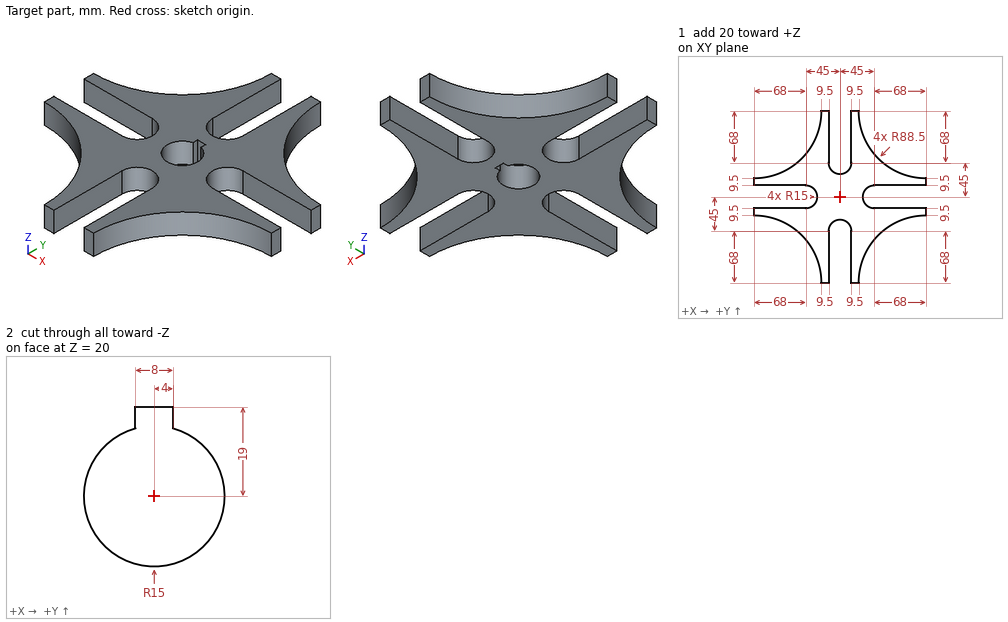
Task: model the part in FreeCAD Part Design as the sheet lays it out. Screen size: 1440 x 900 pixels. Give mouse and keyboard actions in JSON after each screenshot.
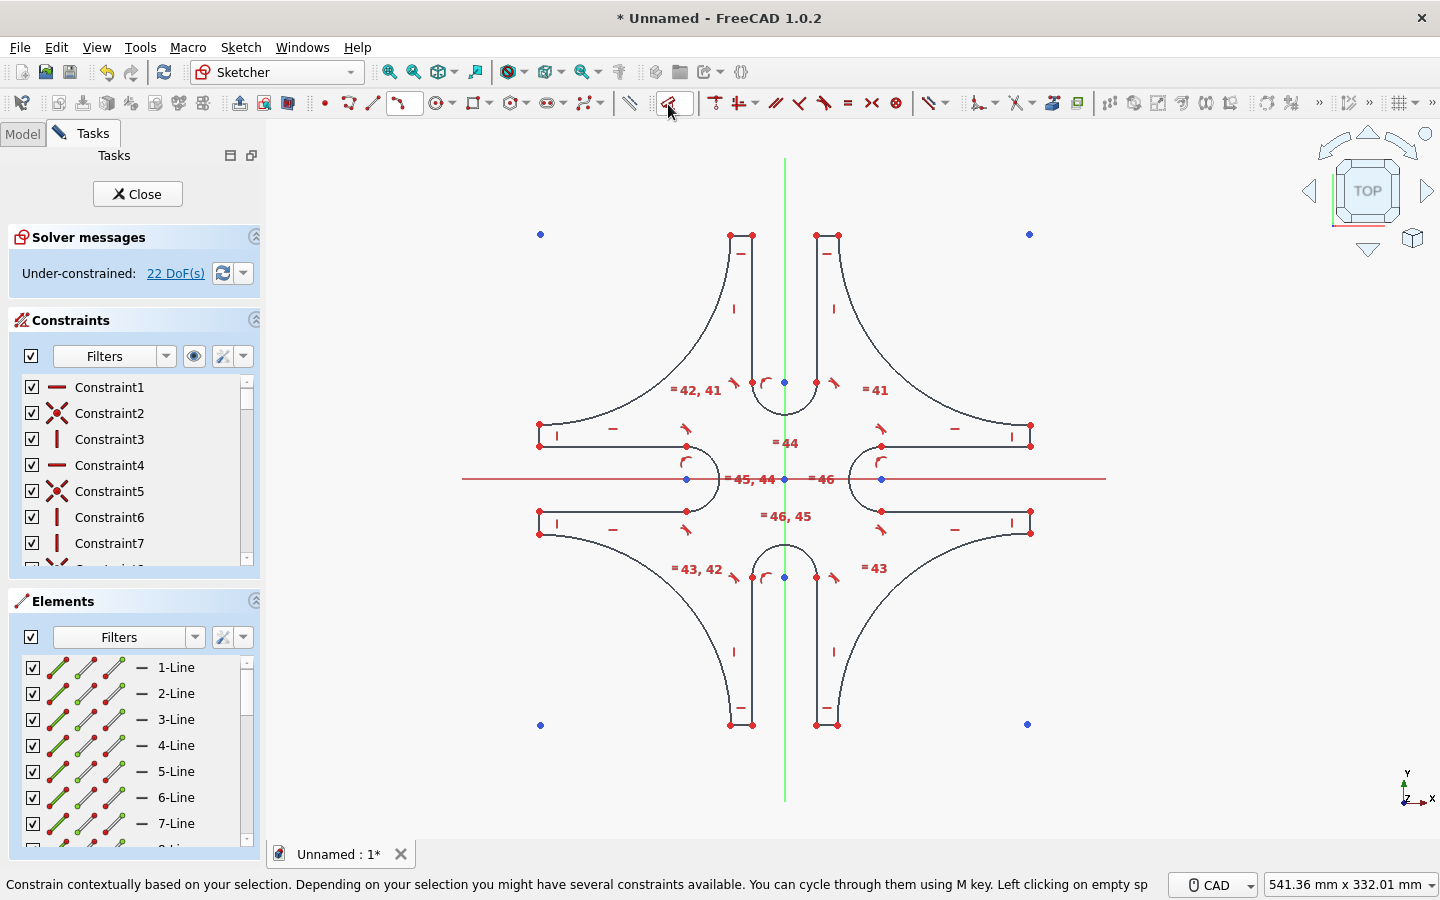
{"action": "left_click", "coordinate": [860, 322]}
{"action": "left_click", "coordinate": [832, 337]}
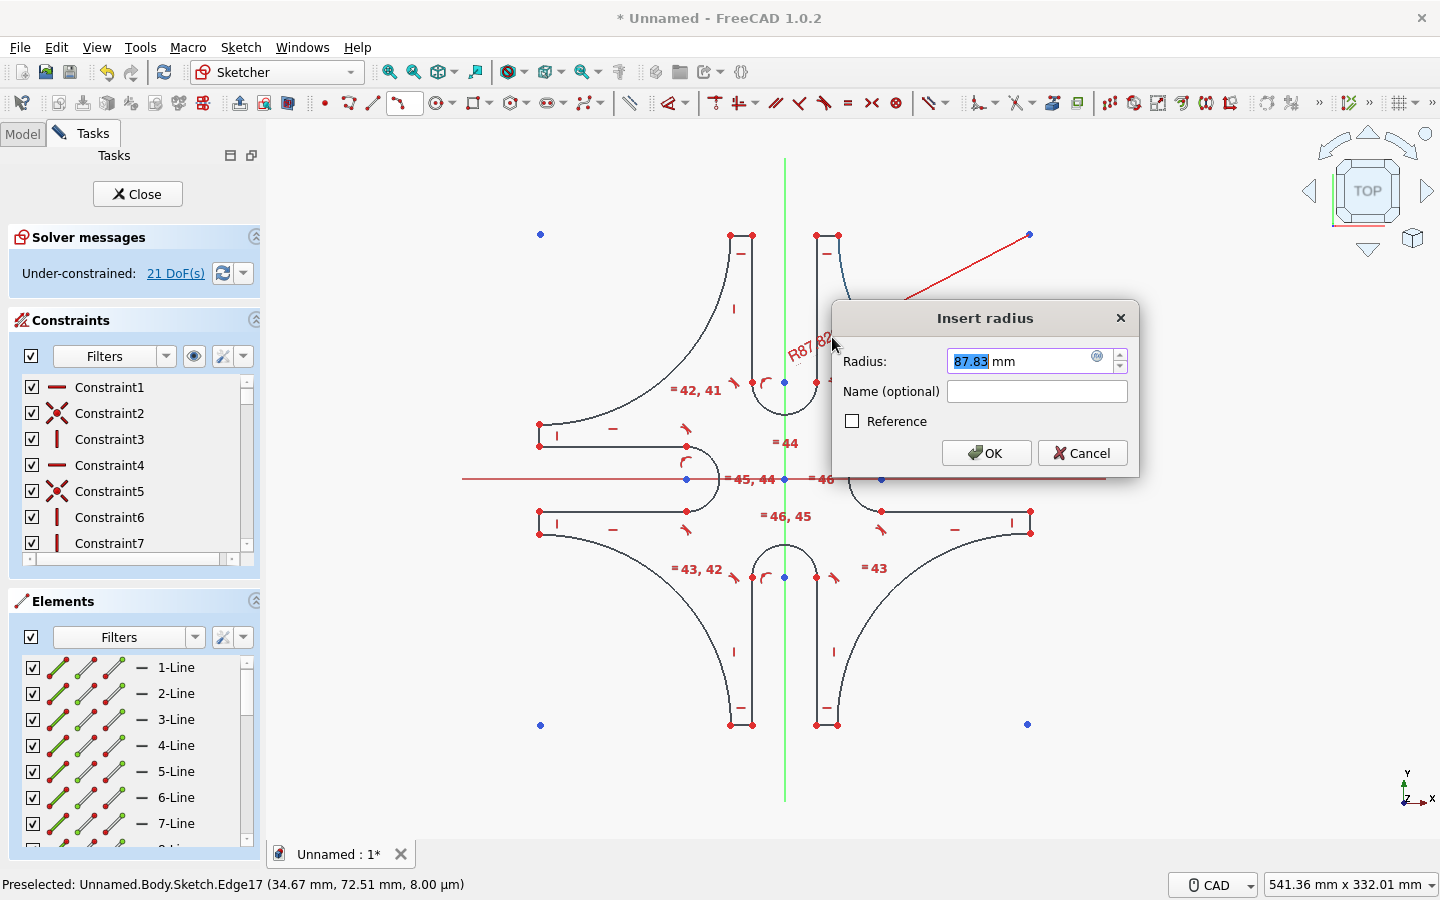
{"action": "type", "text": "88.5"}
{"action": "key", "text": "Return"}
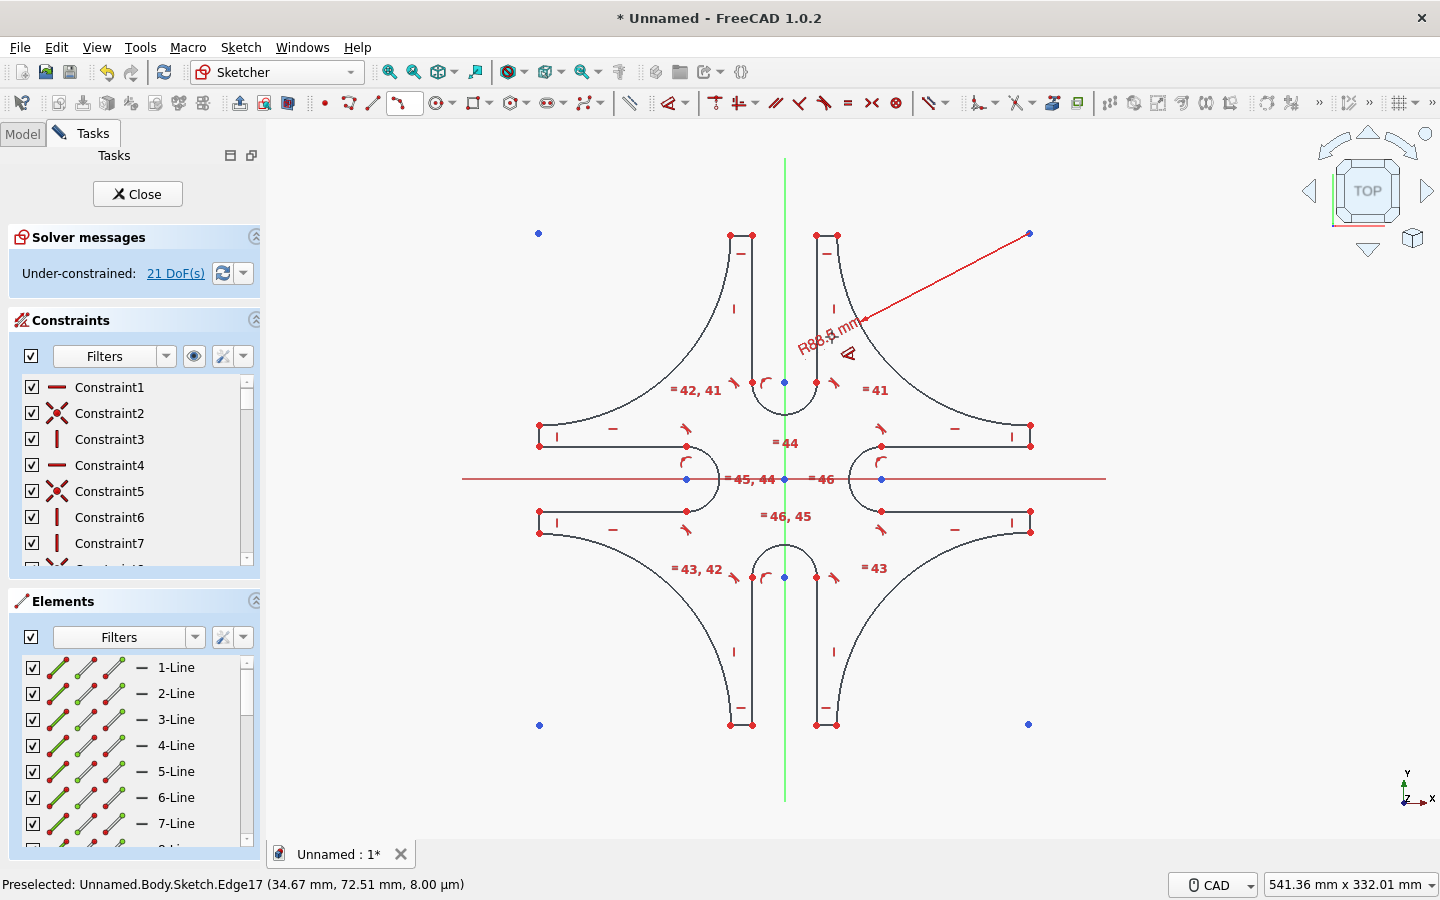
{"action": "left_click", "coordinate": [765, 408]}
{"action": "left_click", "coordinate": [746, 433]}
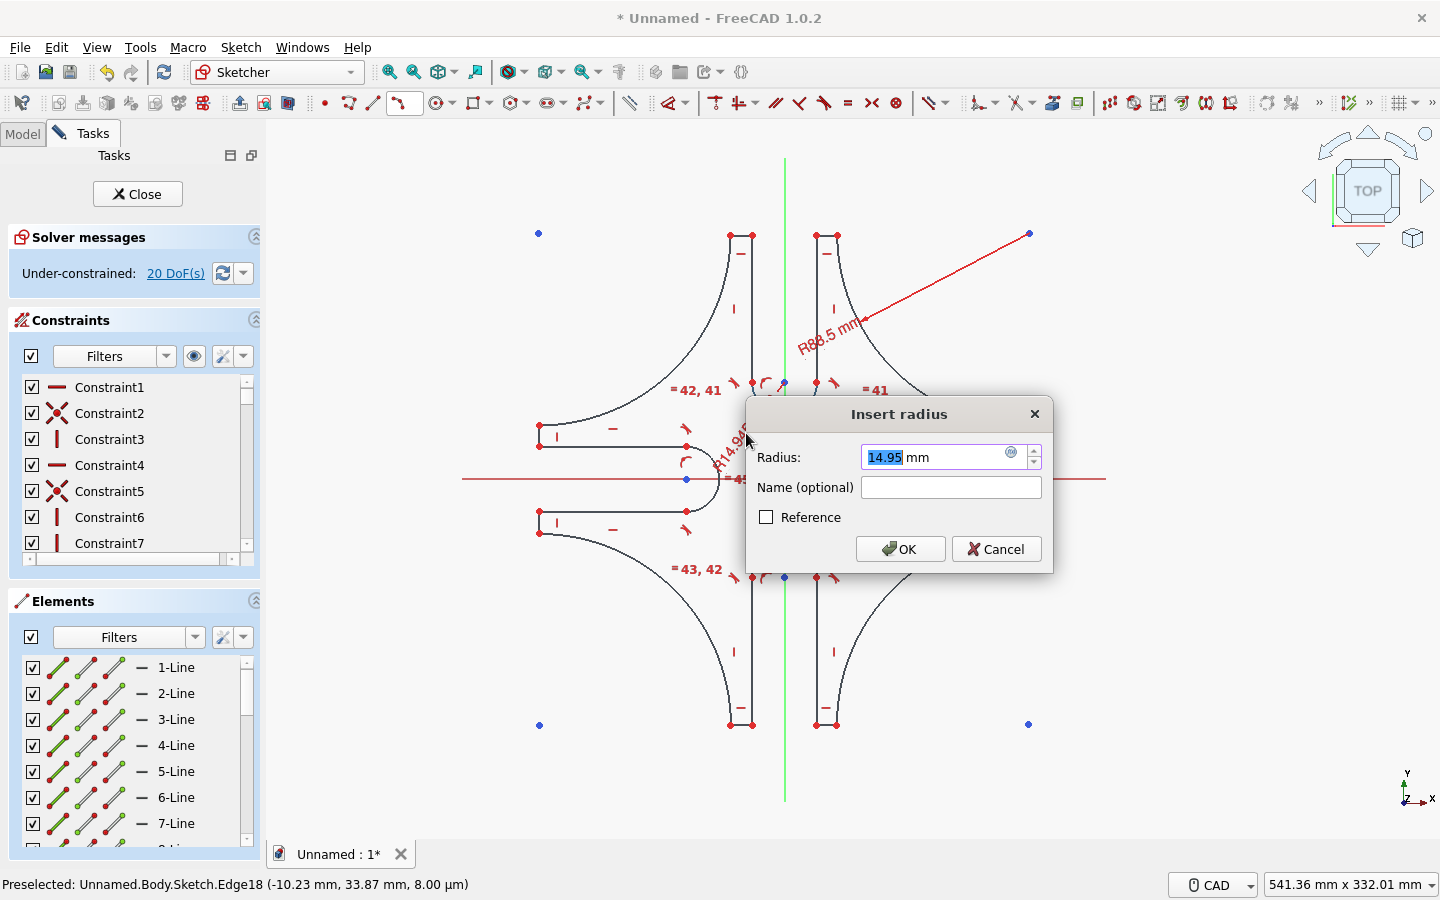
{"action": "type", "text": "15"}
{"action": "key", "text": "Return"}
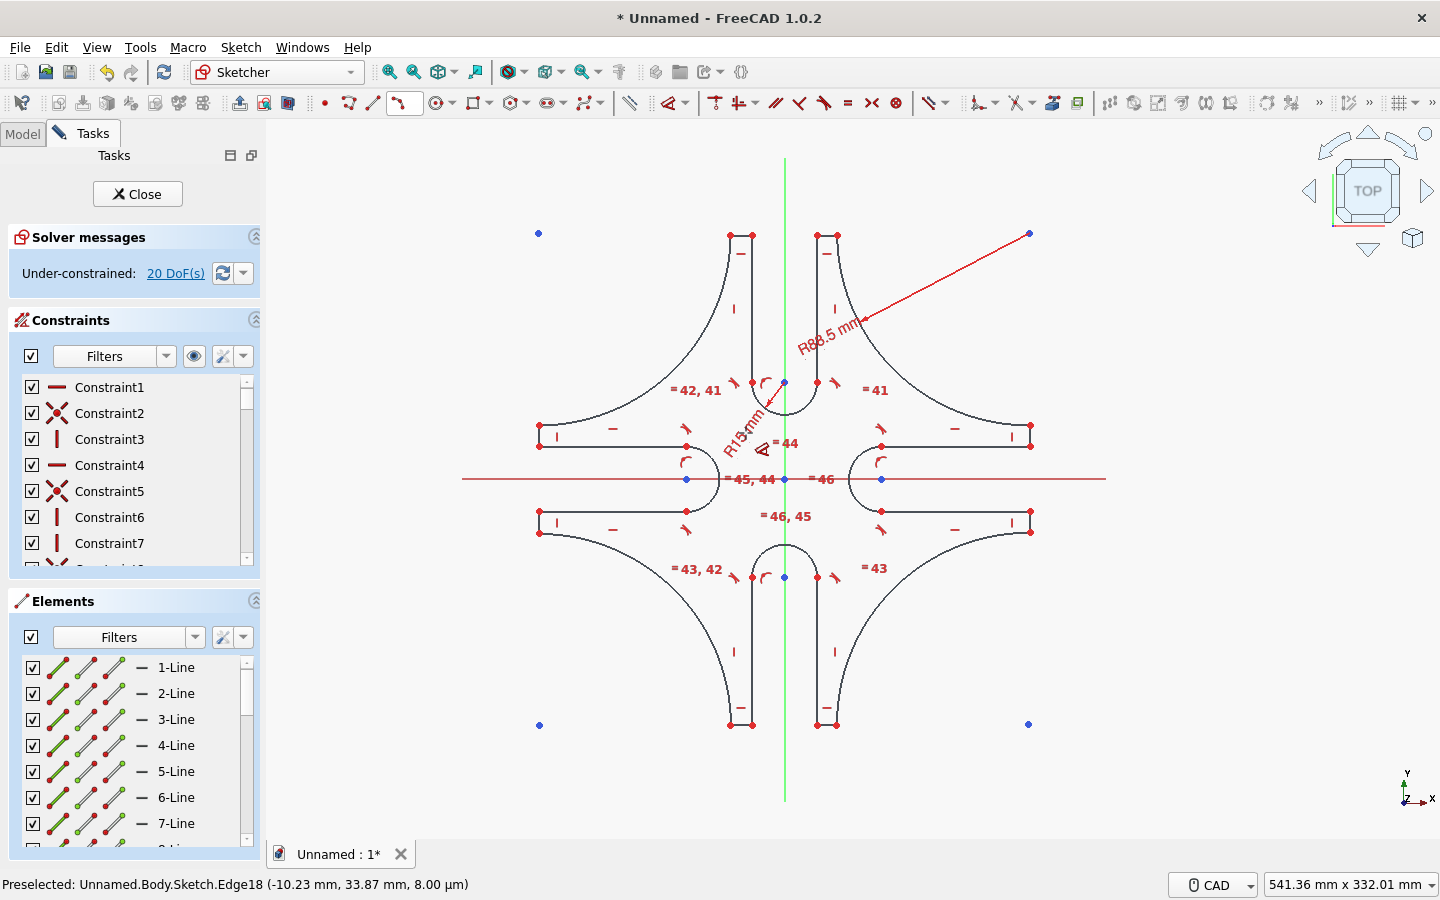
{"action": "left_click", "coordinate": [926, 447]}
{"action": "left_click", "coordinate": [922, 413]}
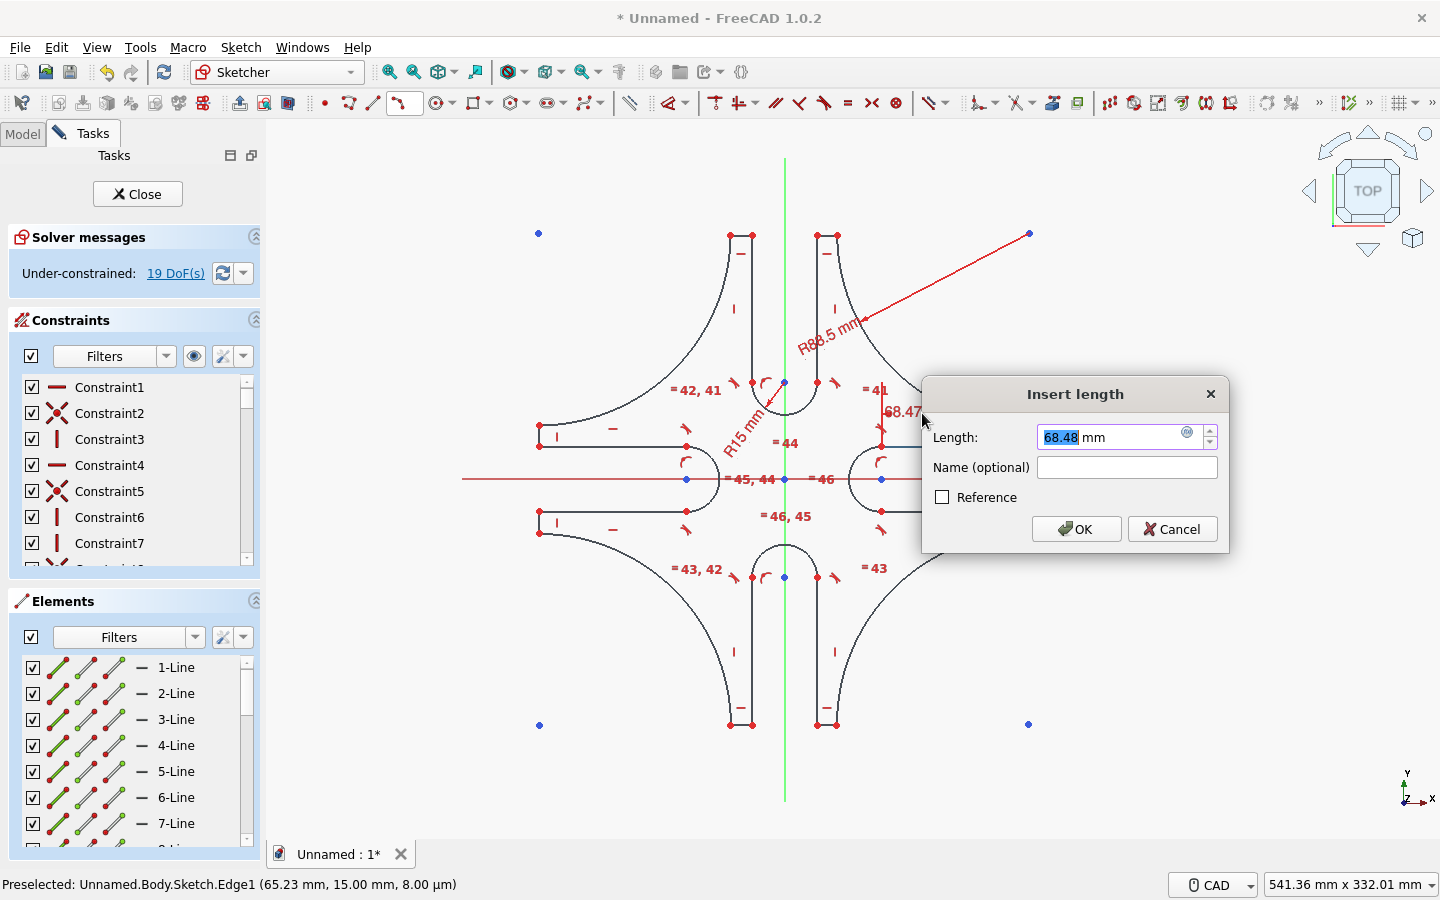
{"action": "type", "text": "68"}
{"action": "key", "text": "Return"}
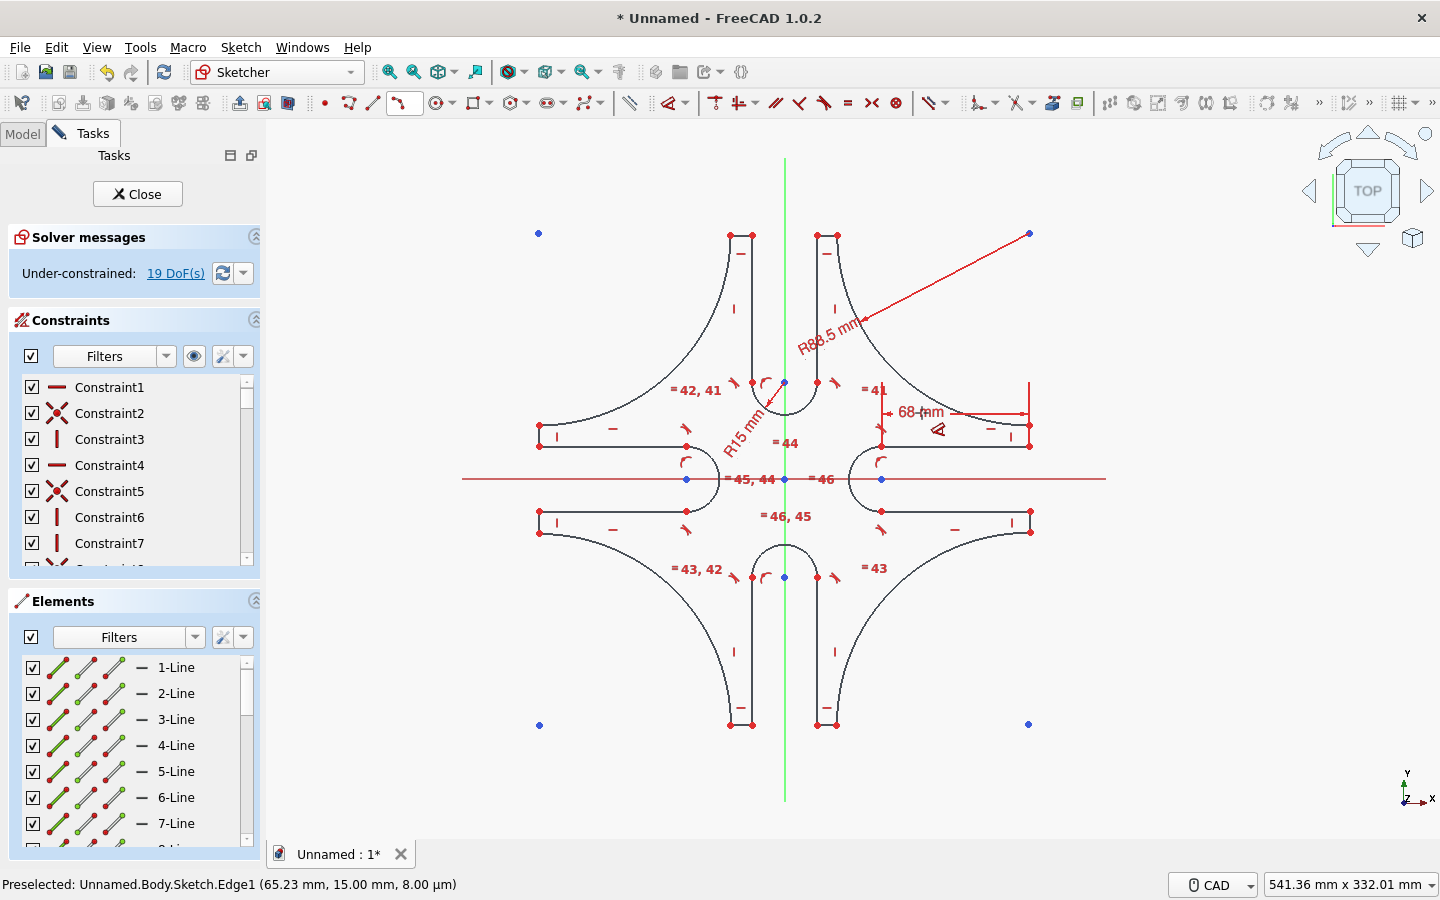
{"action": "left_click", "coordinate": [817, 280]}
{"action": "left_click", "coordinate": [851, 360]}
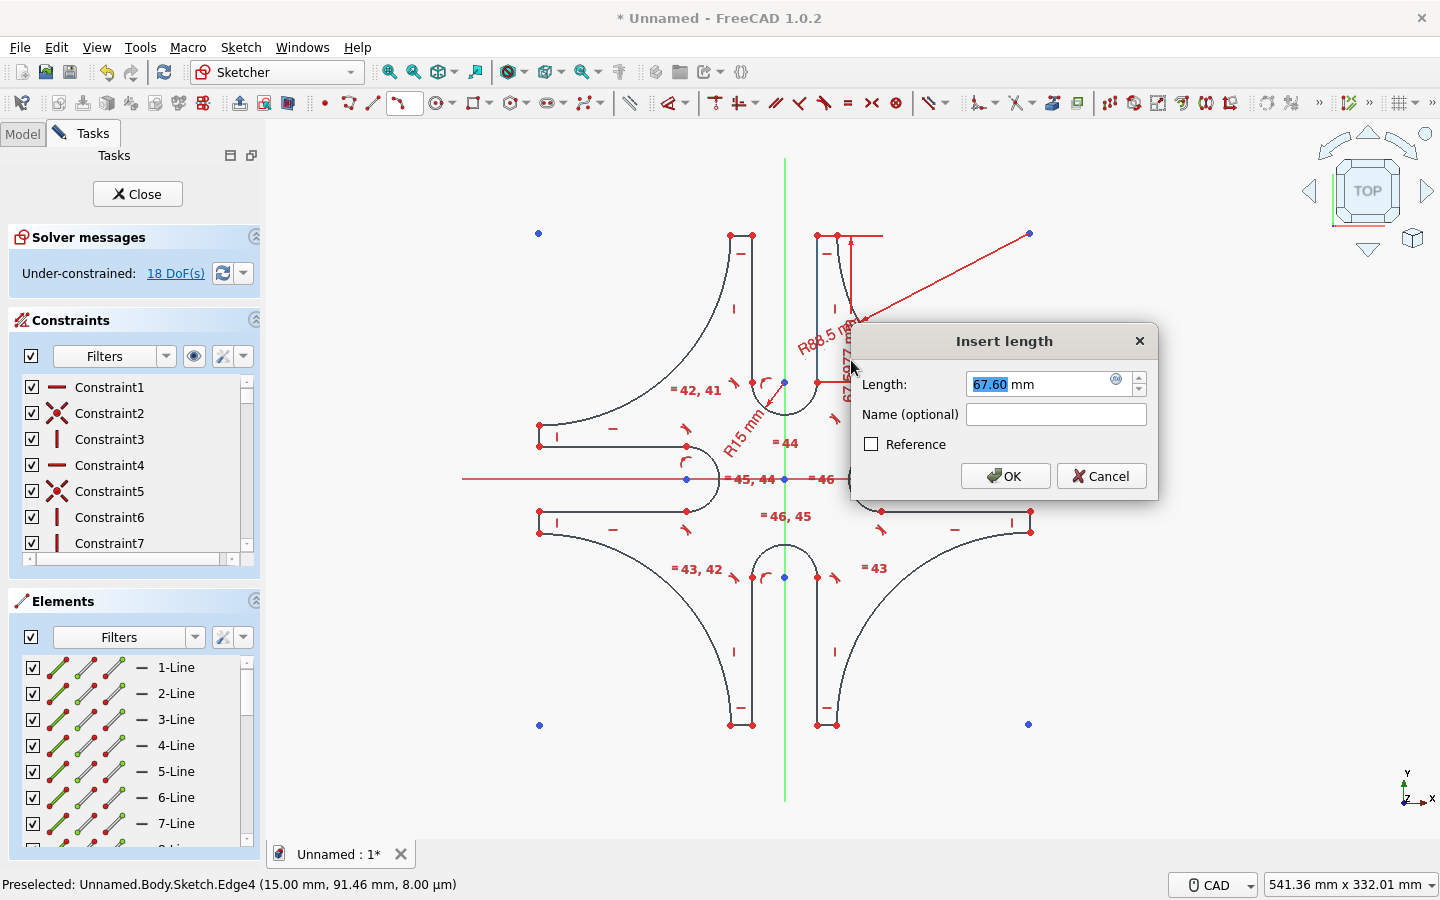
{"action": "type", "text": "68"}
{"action": "key", "text": "Return"}